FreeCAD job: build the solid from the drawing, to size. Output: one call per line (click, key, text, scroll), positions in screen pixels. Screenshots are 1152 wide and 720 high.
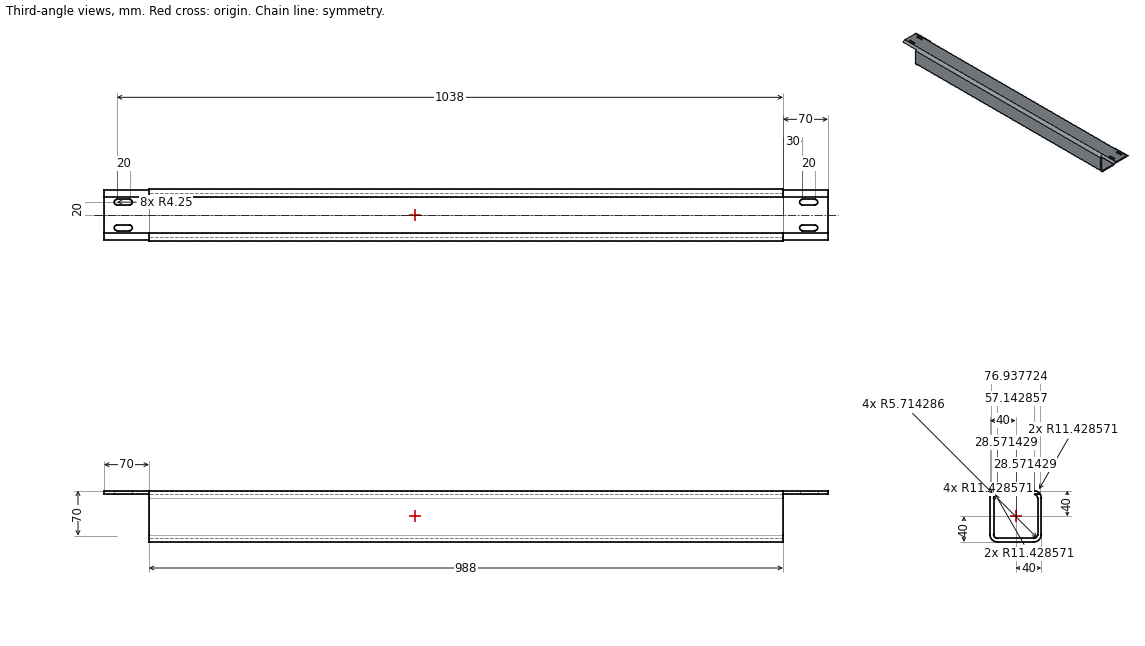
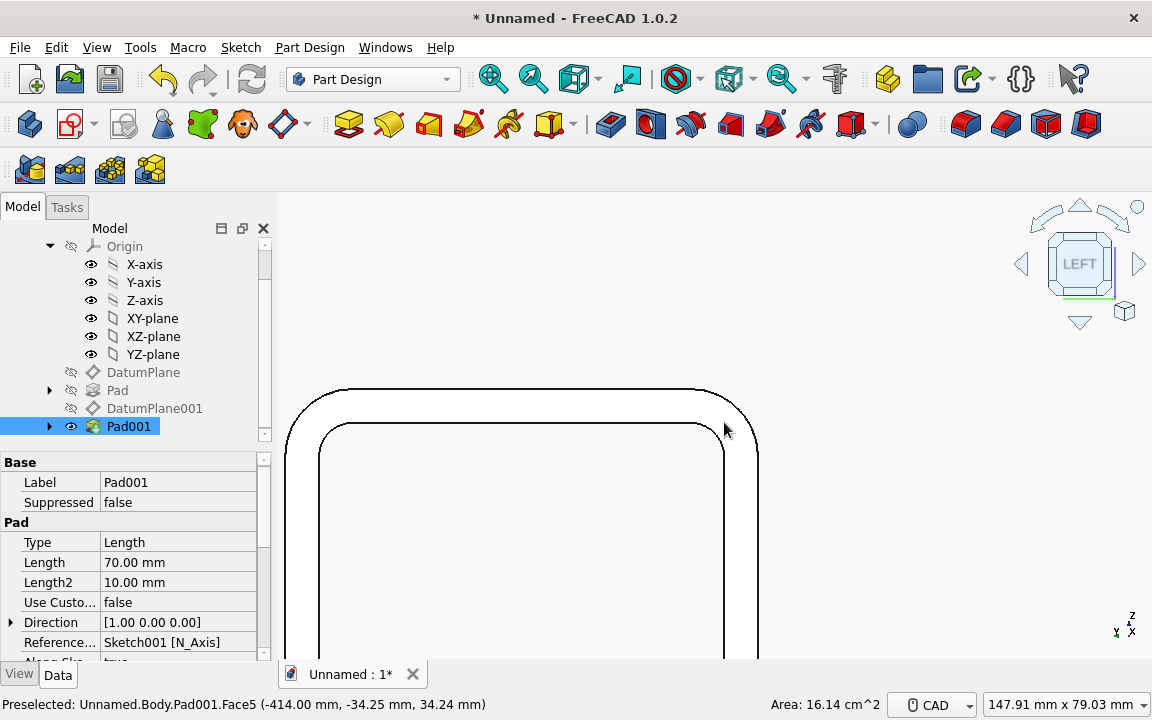
click(70, 124)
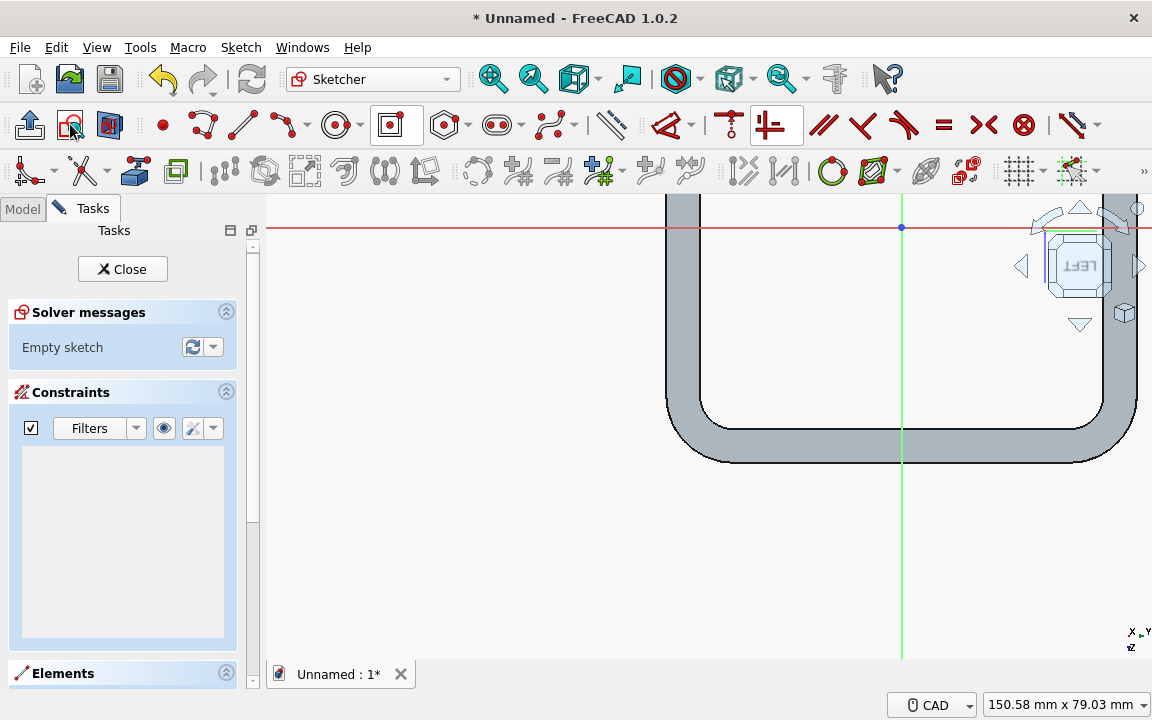
scroll(294, 592, down, 2)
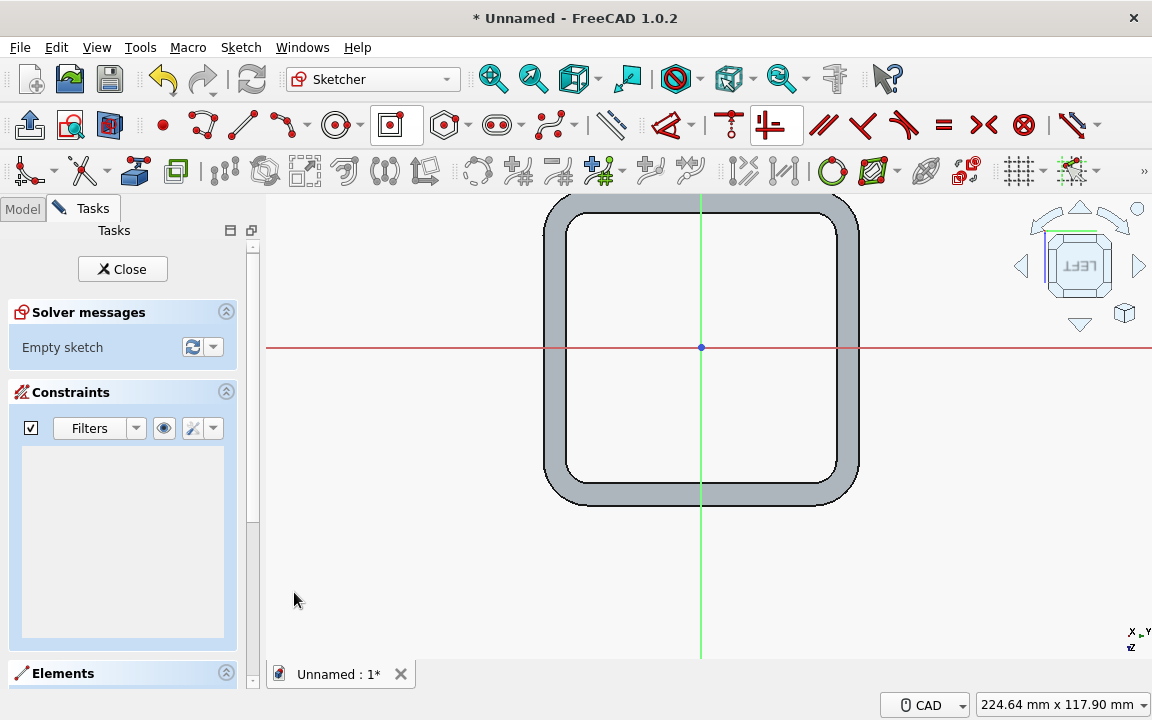
scroll(825, 428, up, 2)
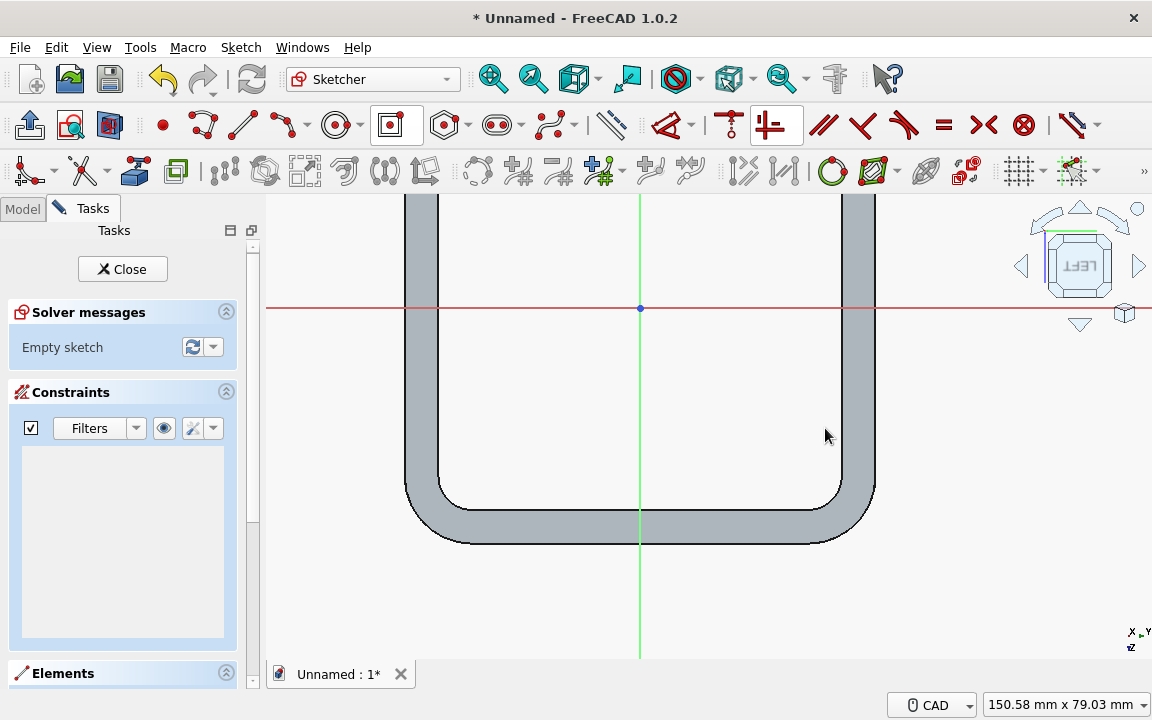
click(244, 126)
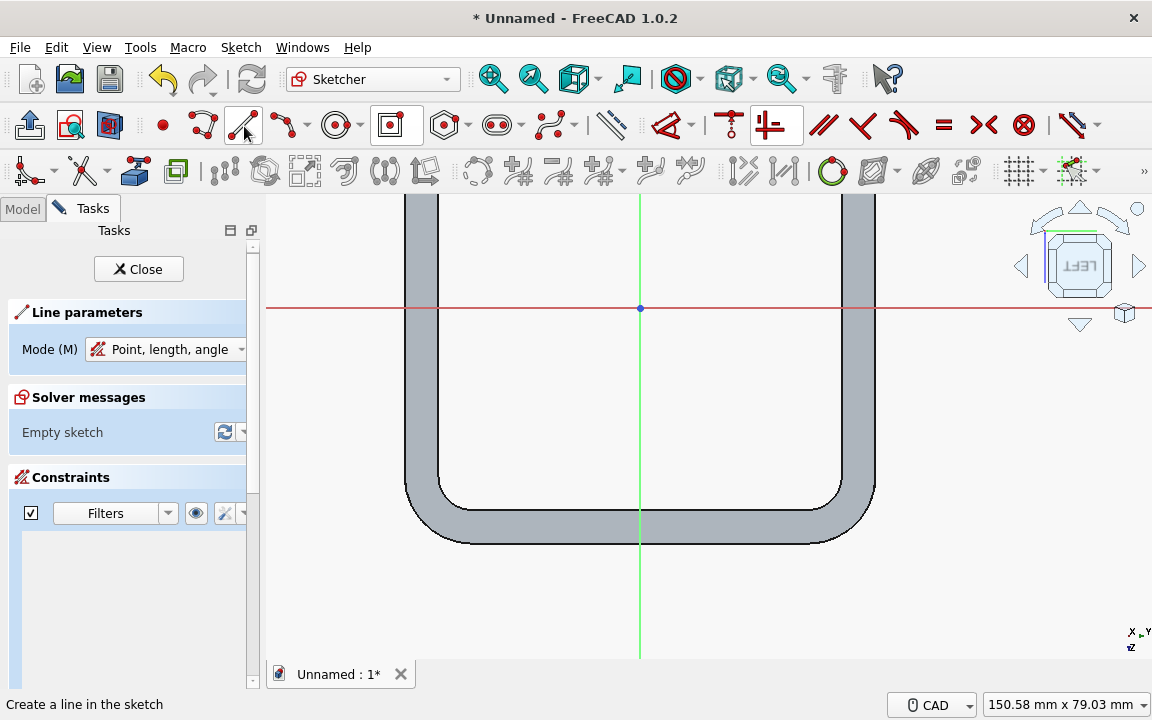
click(472, 544)
click(808, 544)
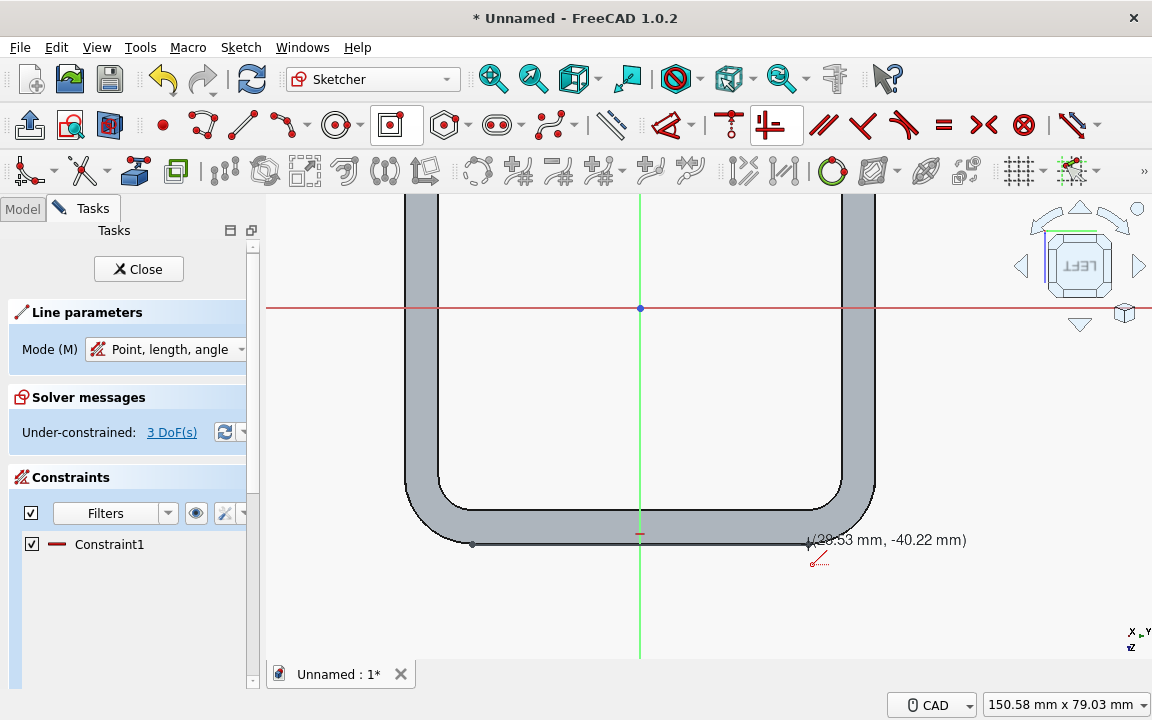
click(866, 510)
click(414, 510)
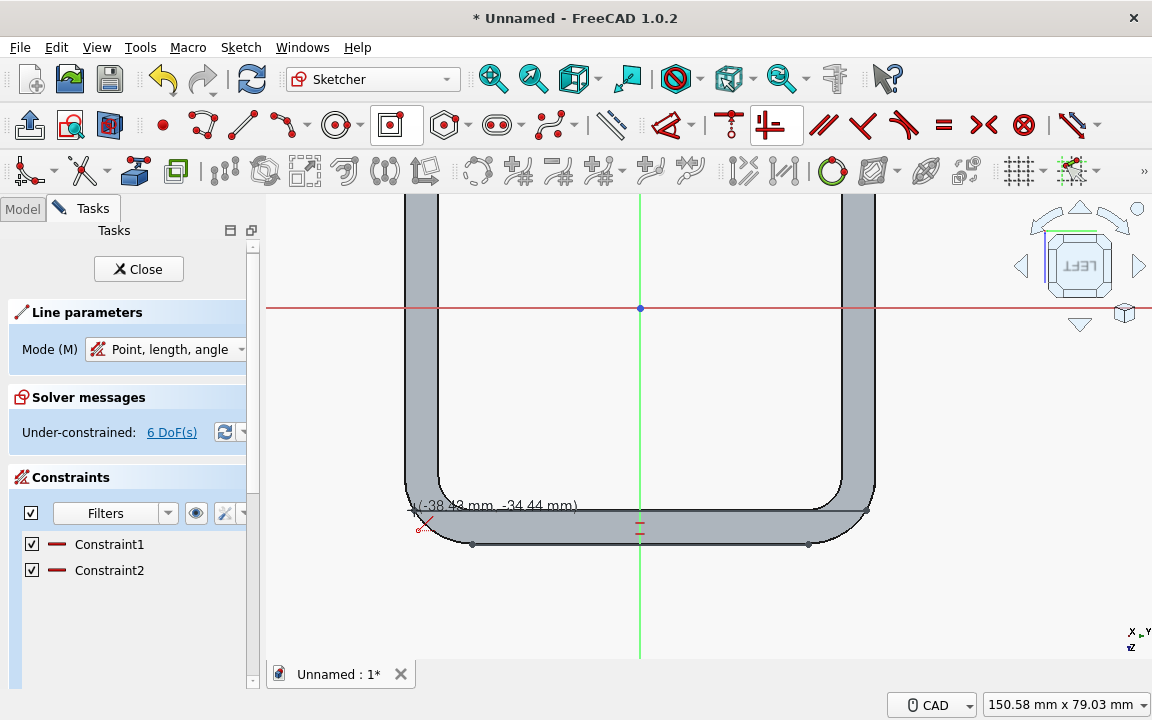
key(g)
key(3)
key(a)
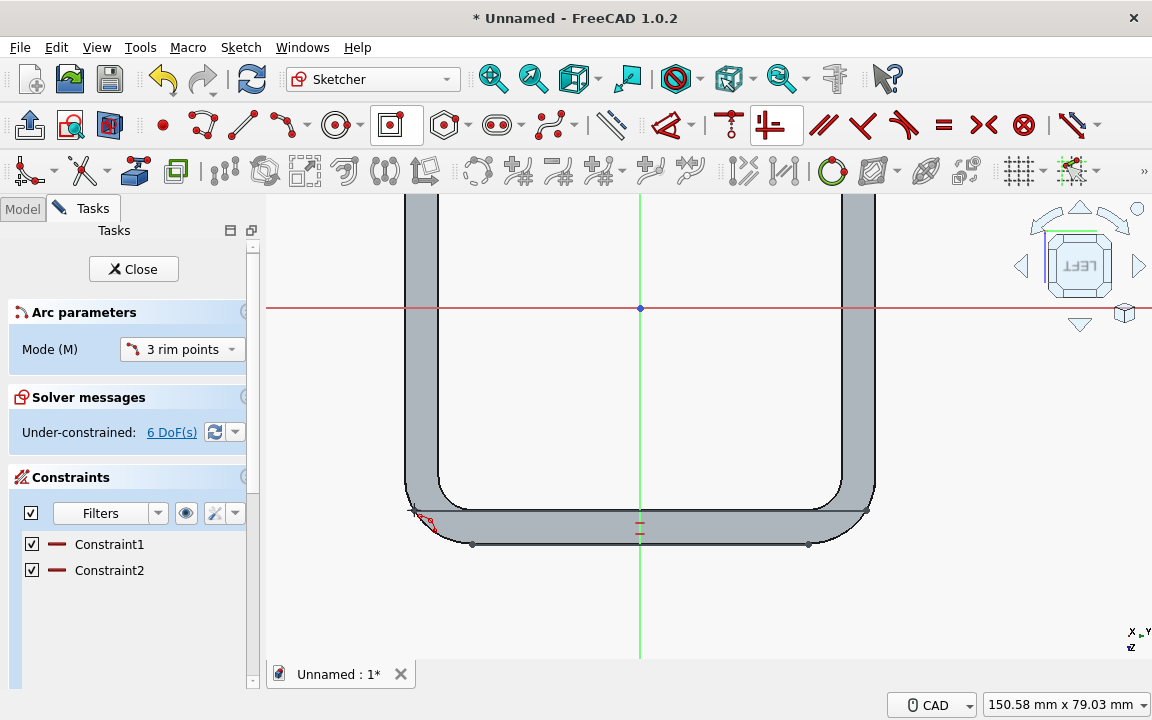
click(808, 545)
click(866, 511)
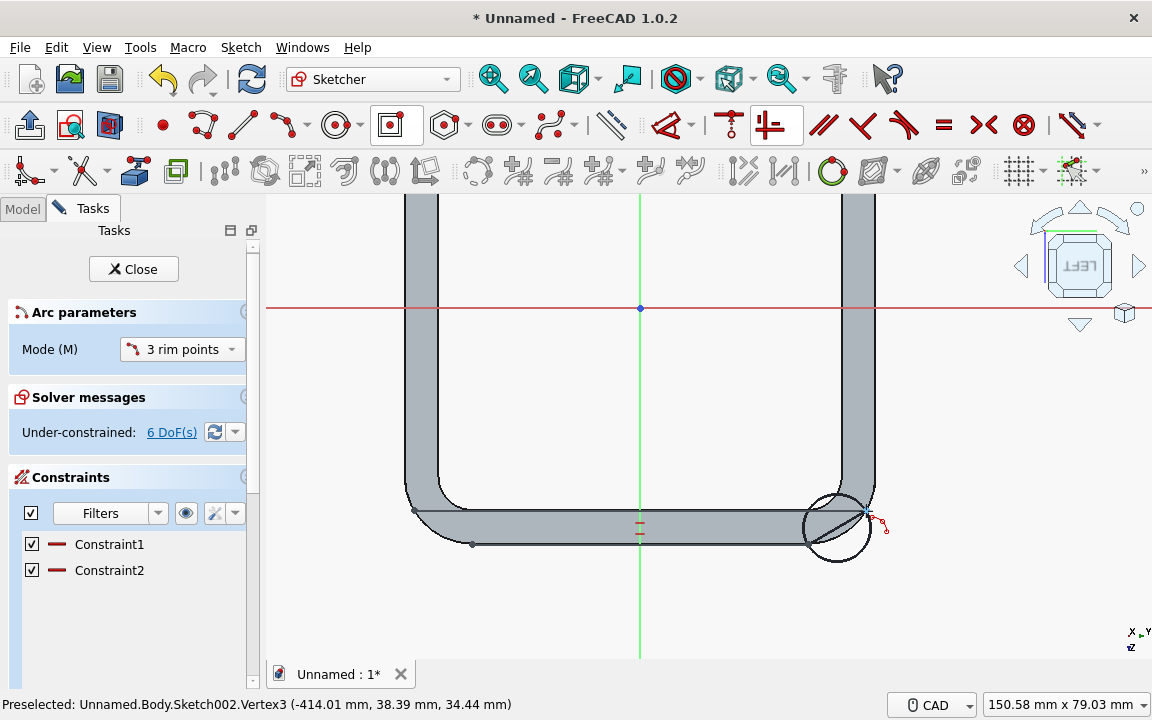
scroll(842, 535, up, 3)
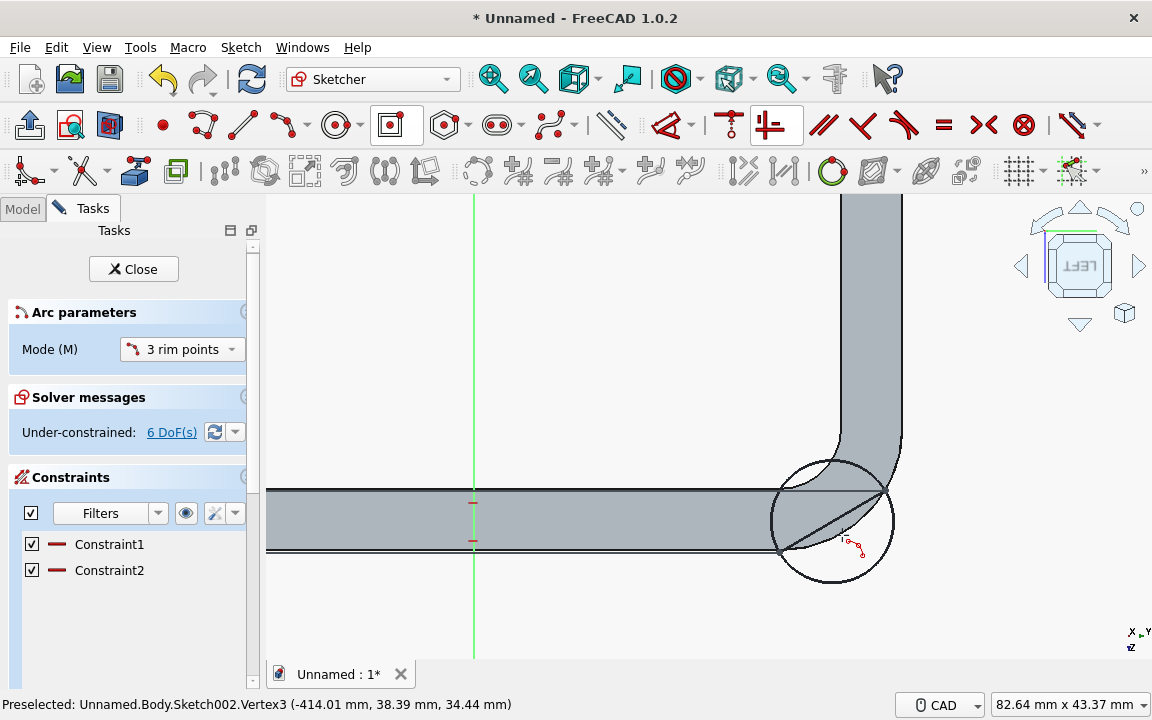
click(841, 534)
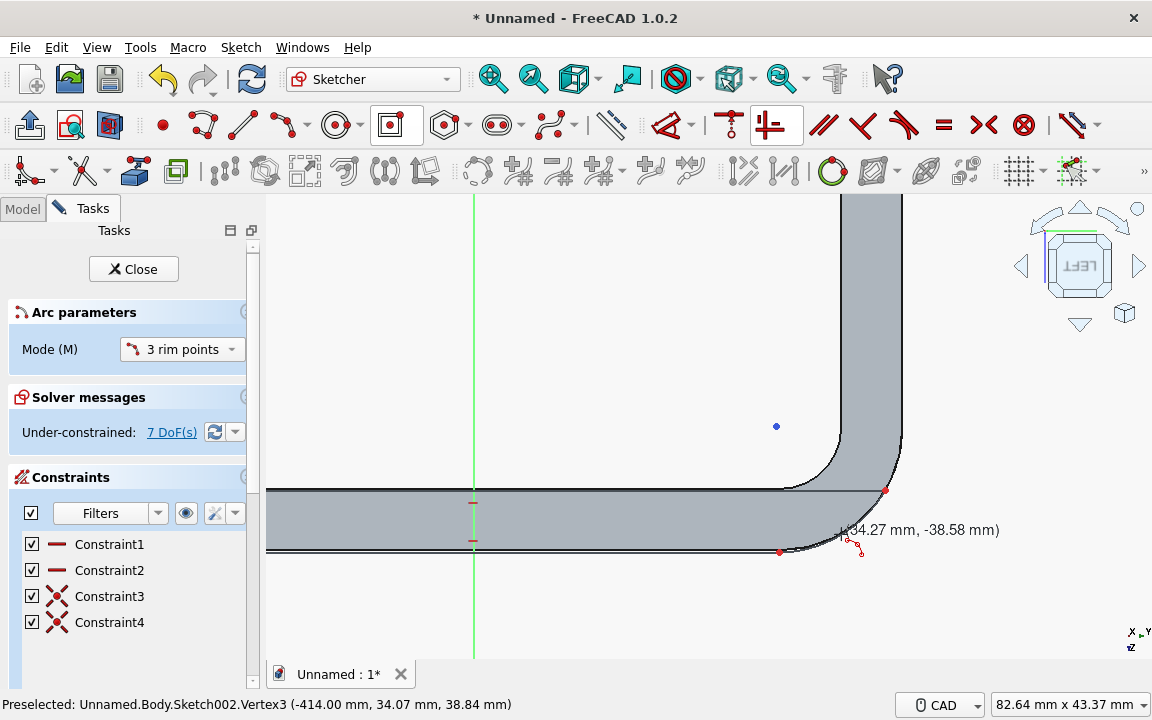
scroll(843, 537, down, 3)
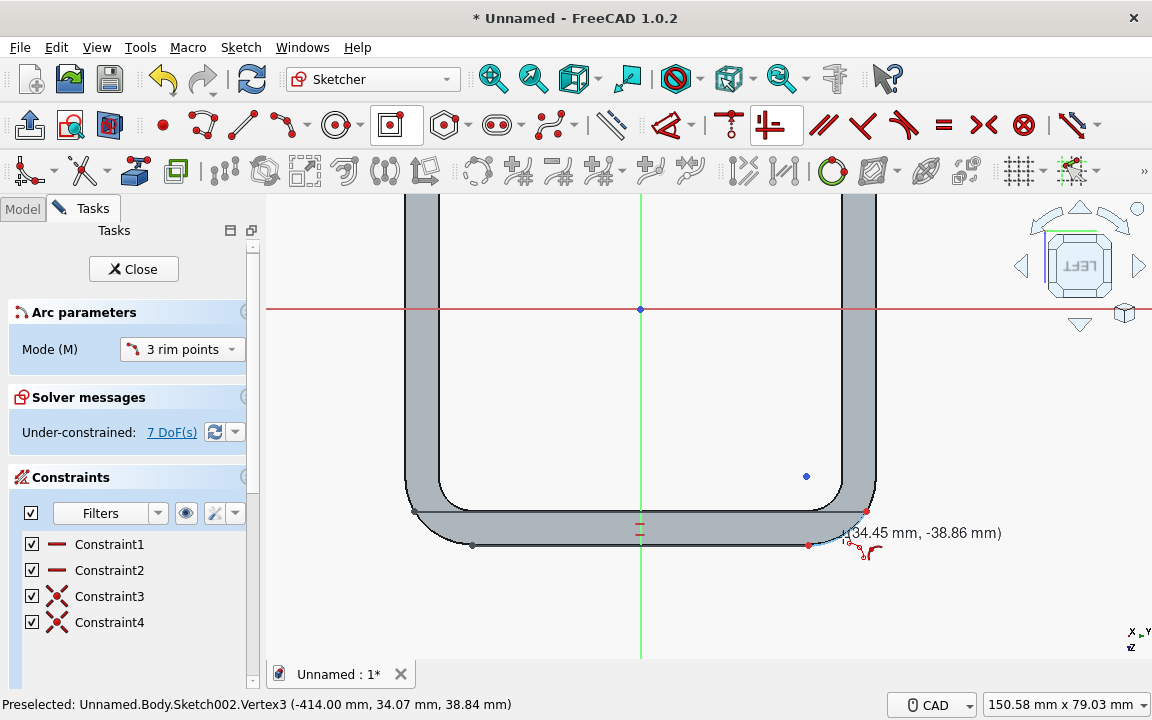
click(414, 512)
click(472, 546)